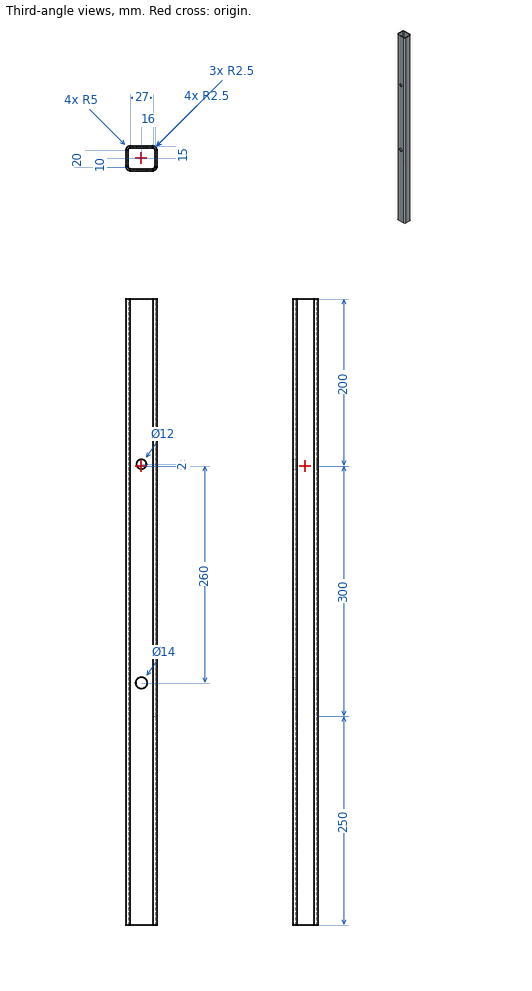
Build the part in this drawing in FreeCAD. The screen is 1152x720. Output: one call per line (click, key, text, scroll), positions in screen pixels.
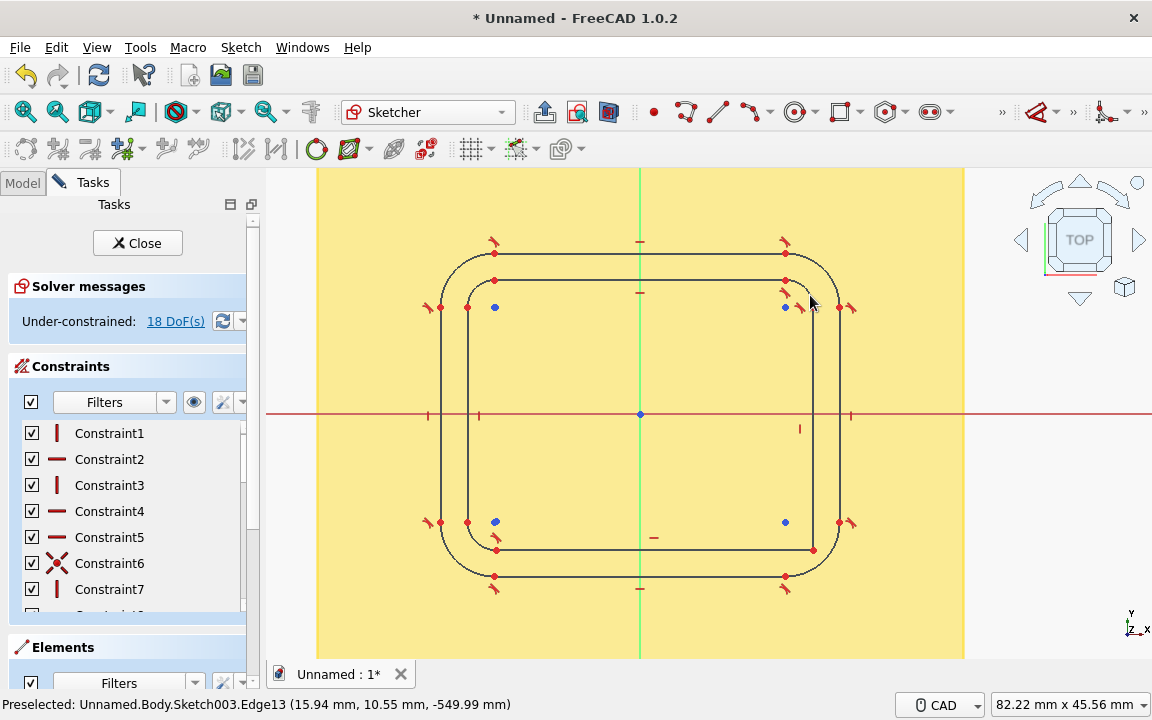
click(699, 280)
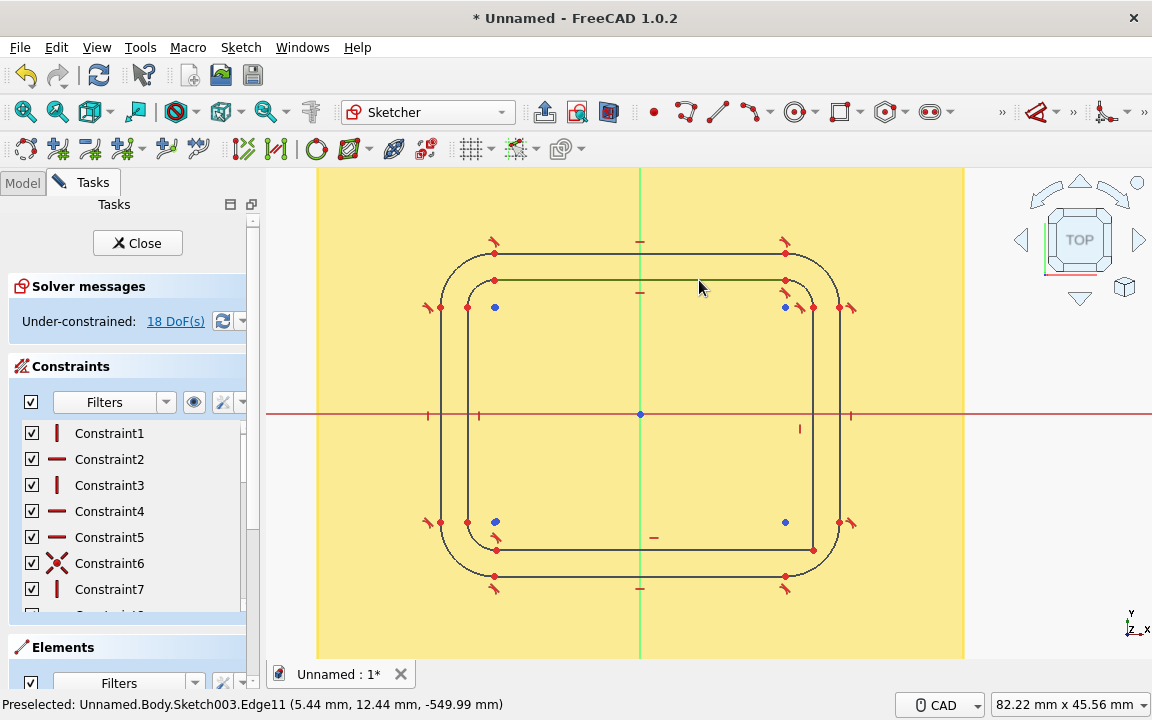
click(482, 283)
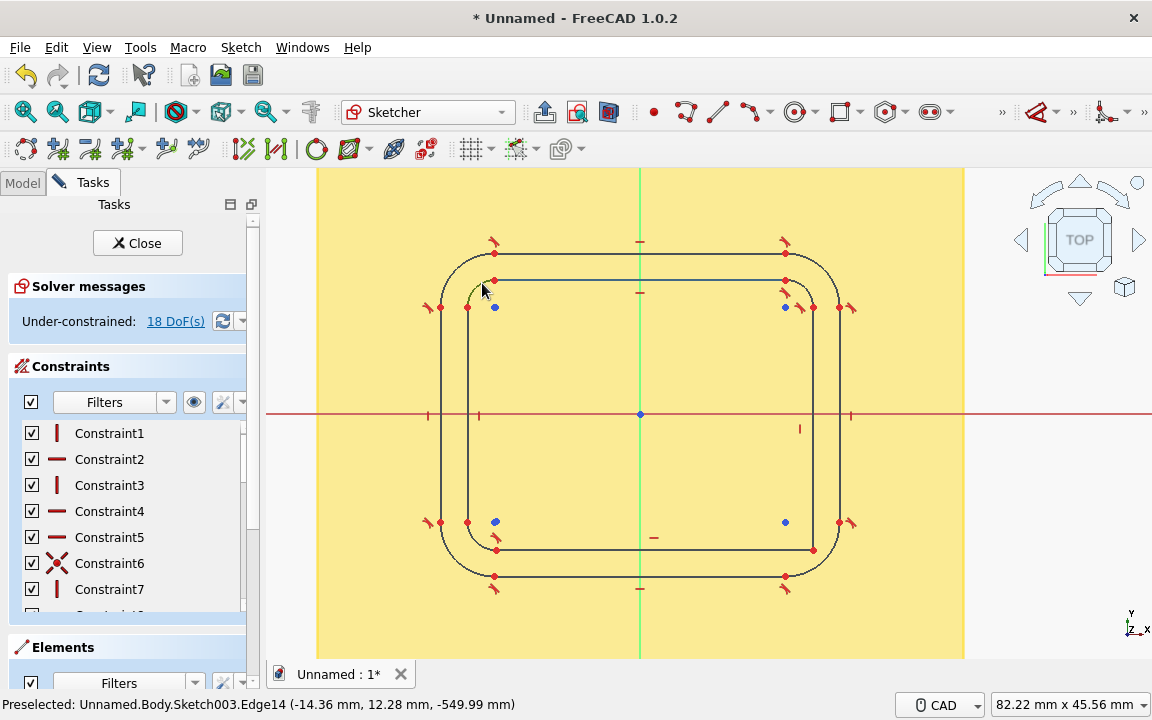
key(t)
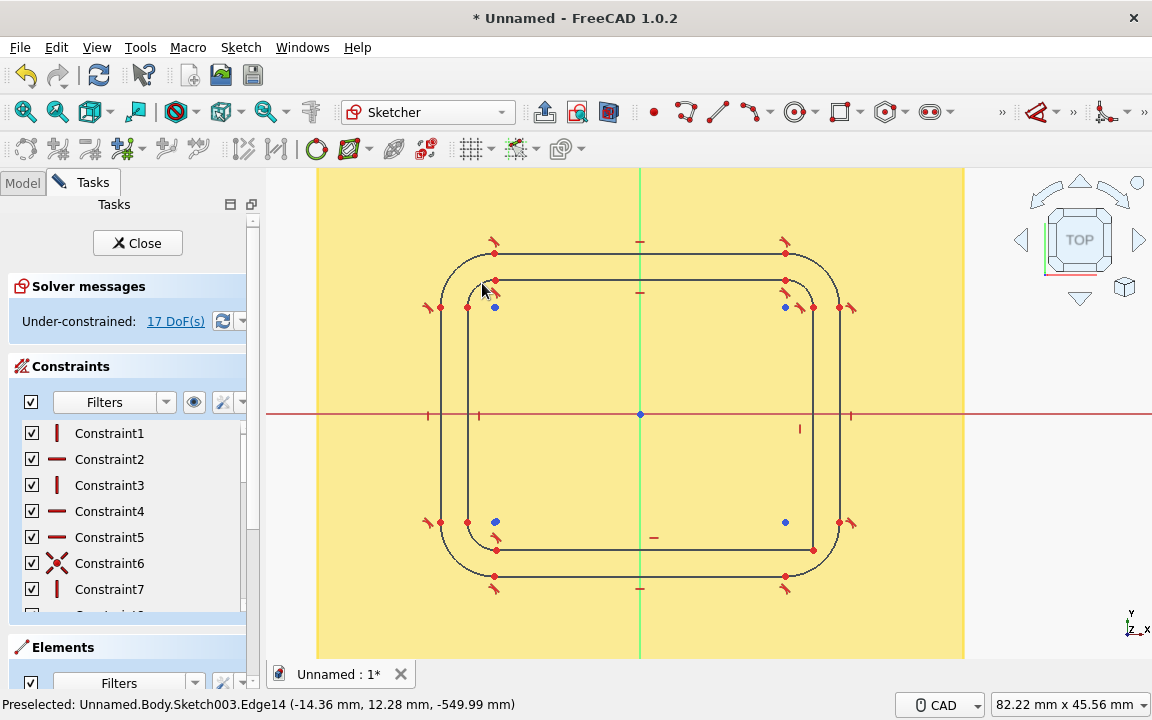
click(468, 372)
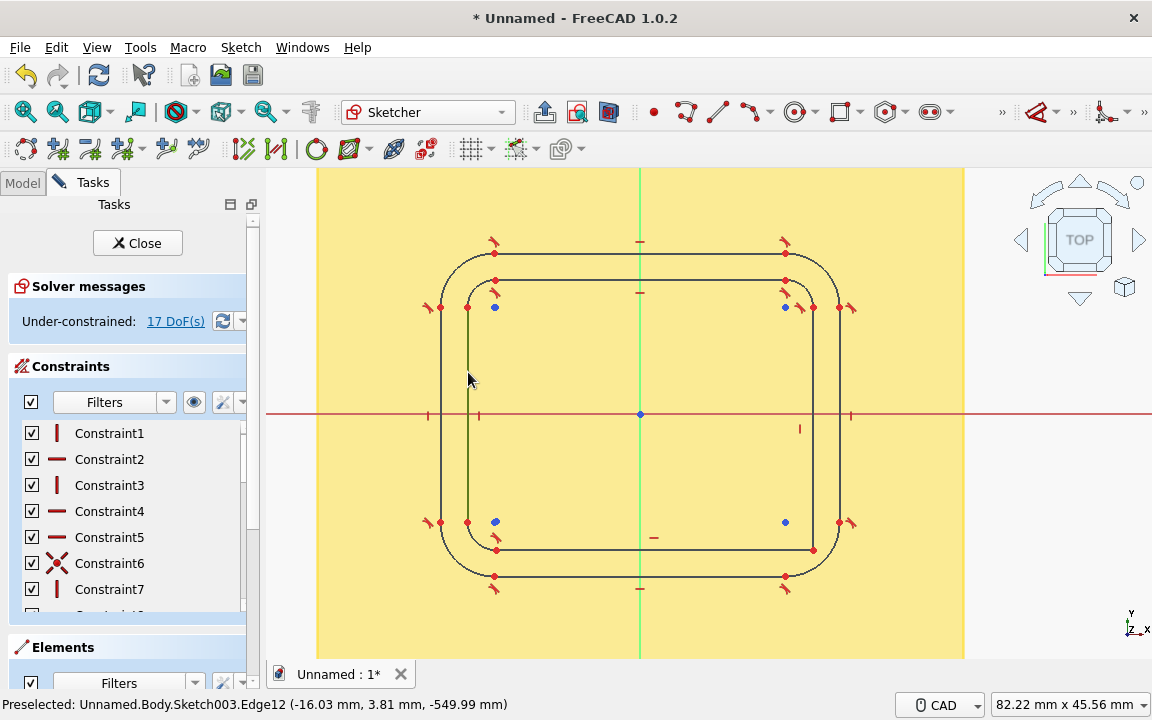
click(483, 283)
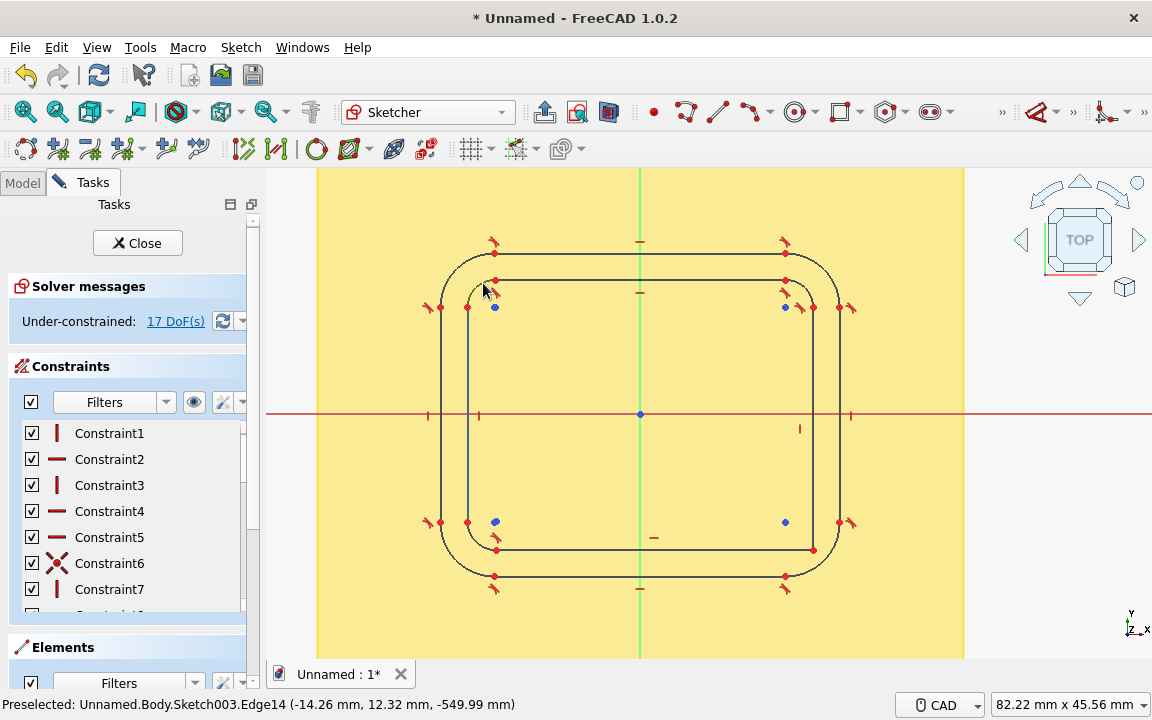
key(t)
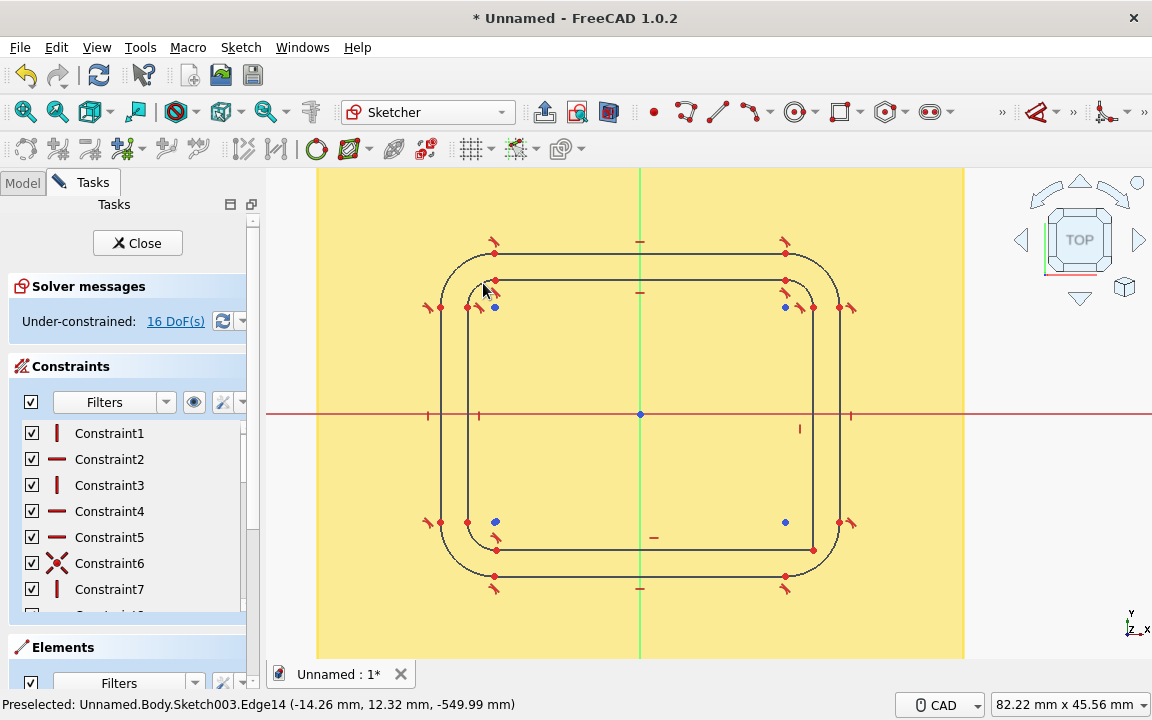
click(468, 372)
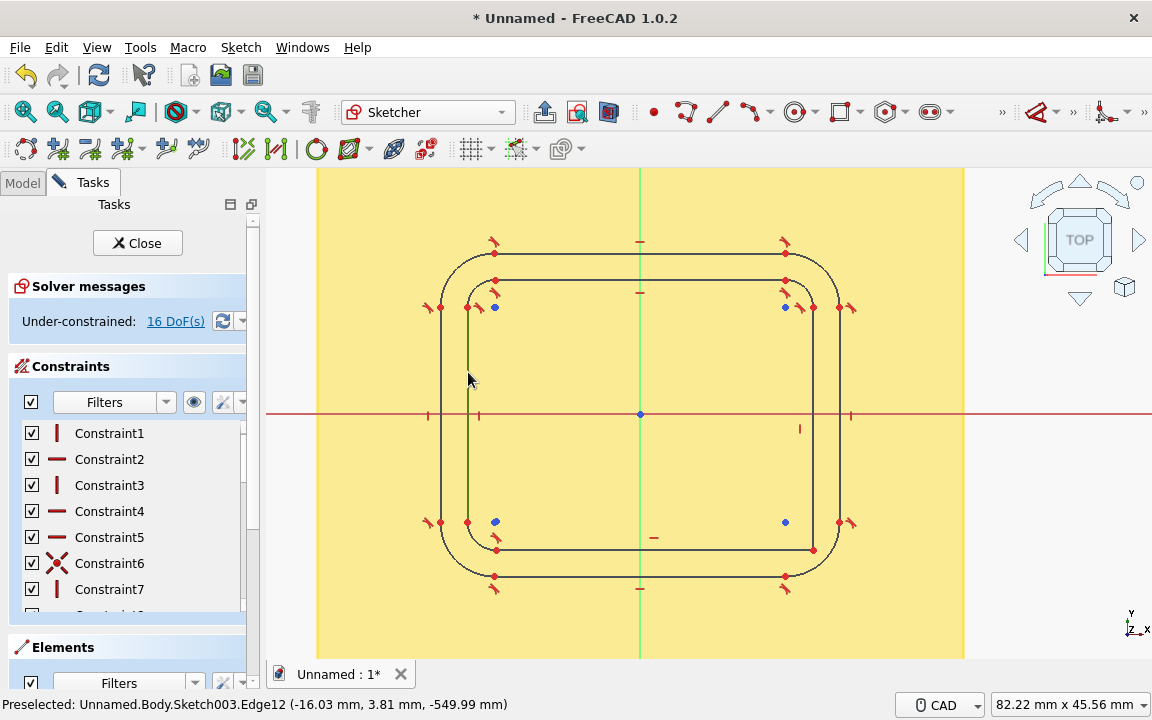
click(471, 535)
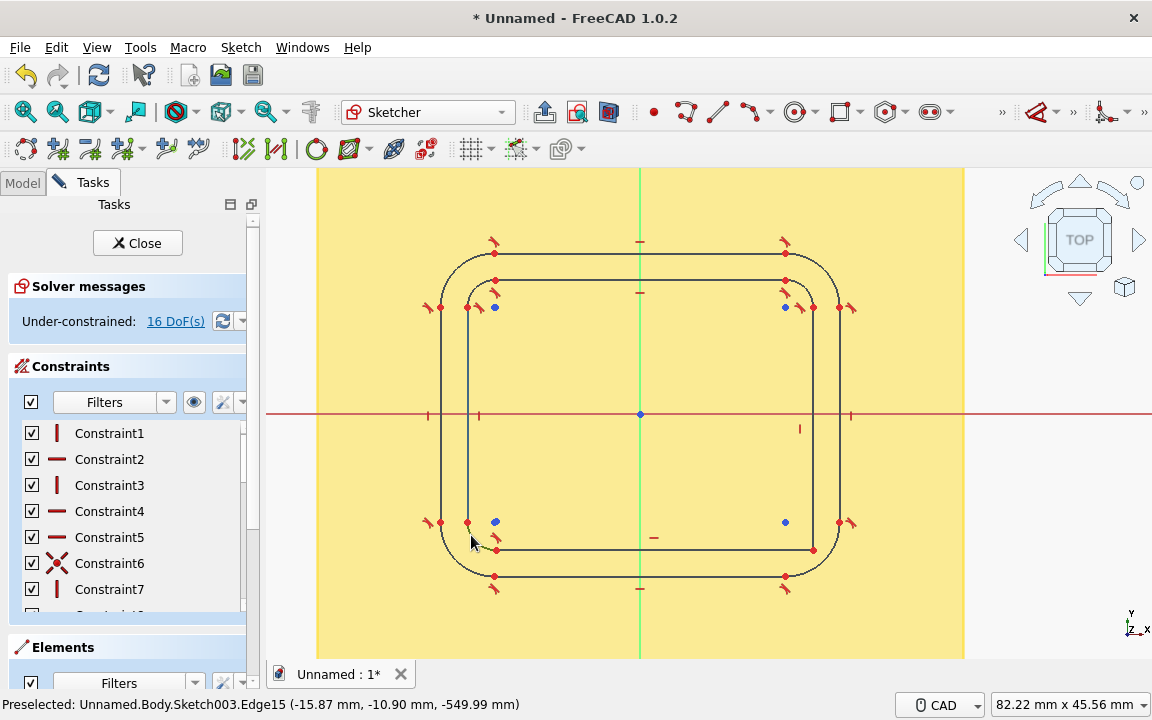
key(t)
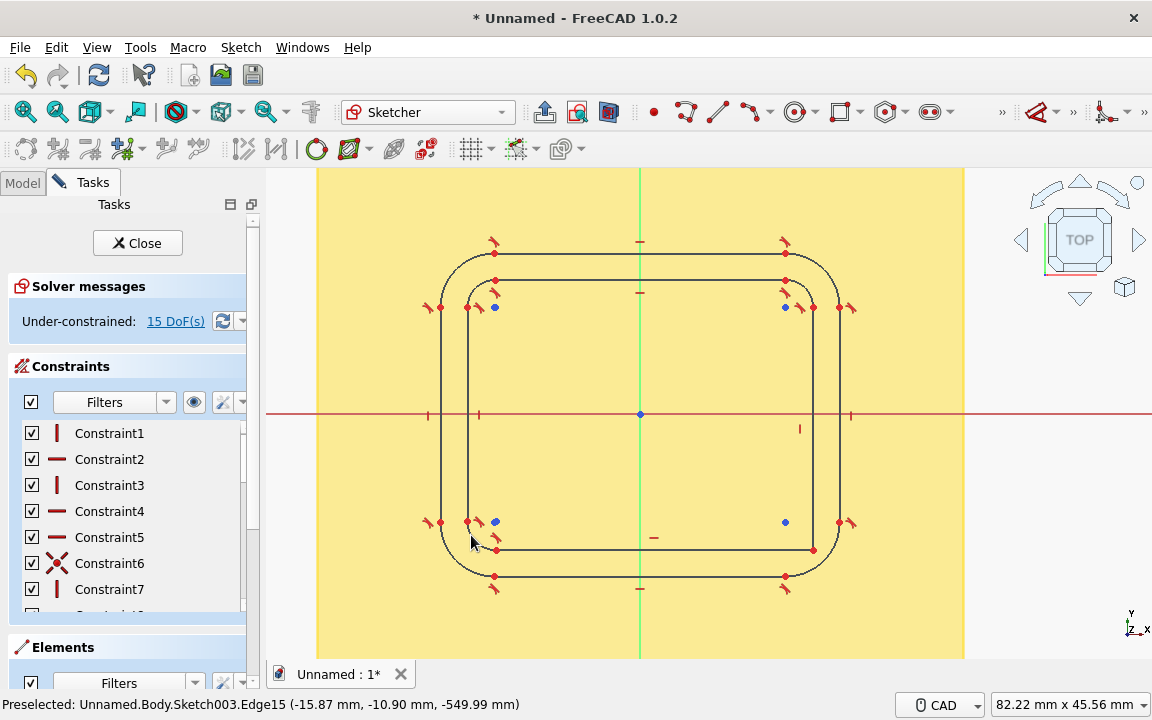
click(834, 283)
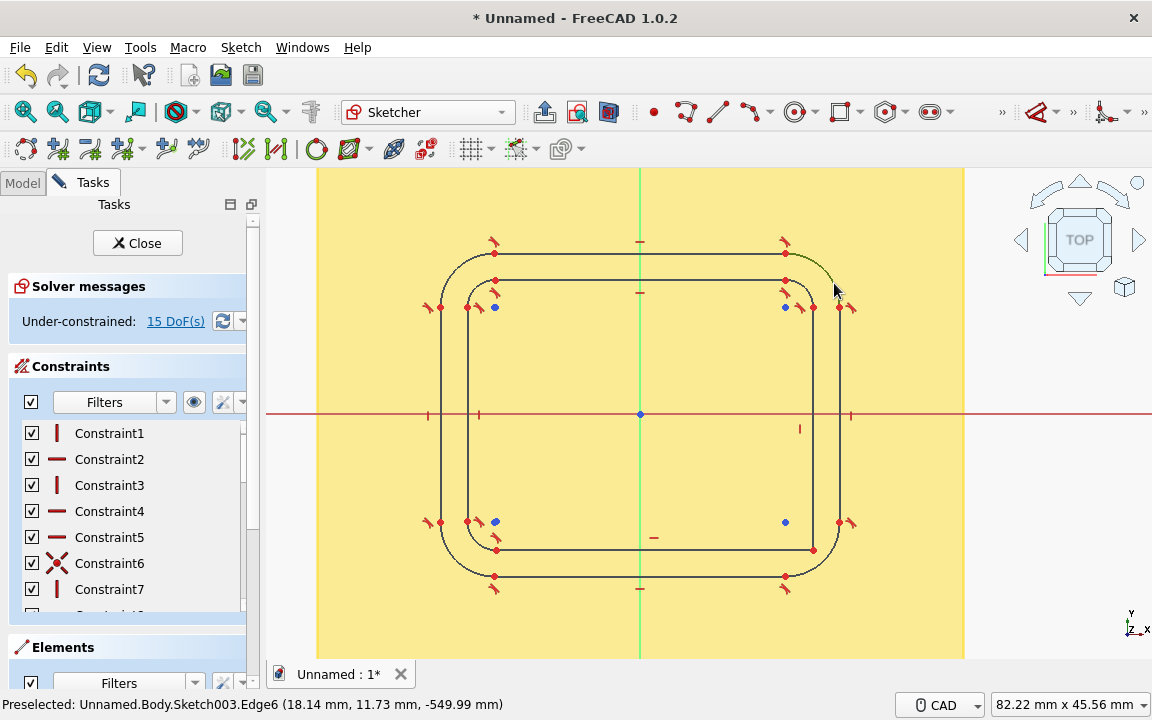
click(810, 295)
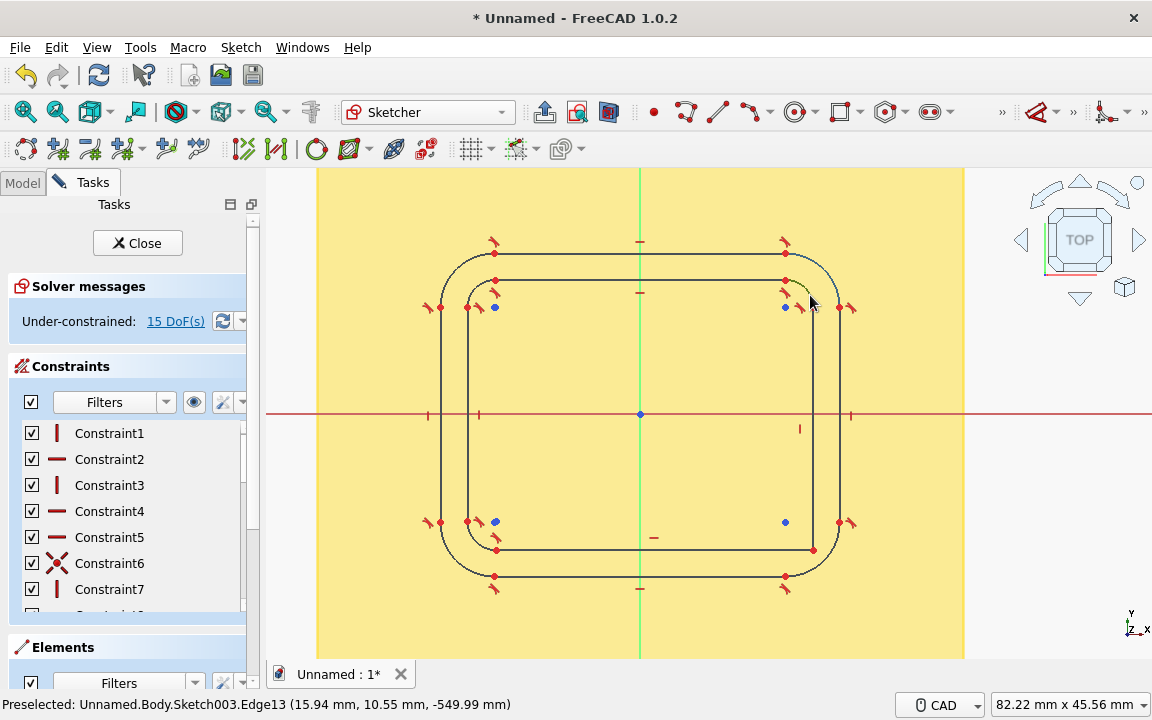
key(c)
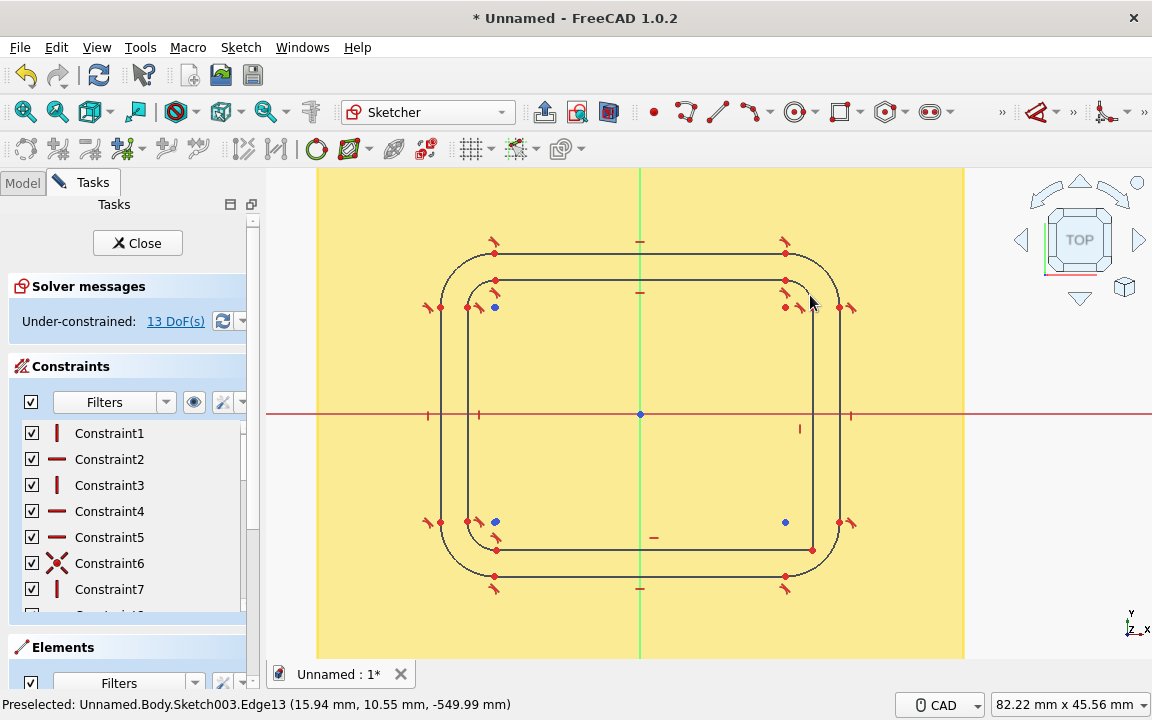
click(470, 259)